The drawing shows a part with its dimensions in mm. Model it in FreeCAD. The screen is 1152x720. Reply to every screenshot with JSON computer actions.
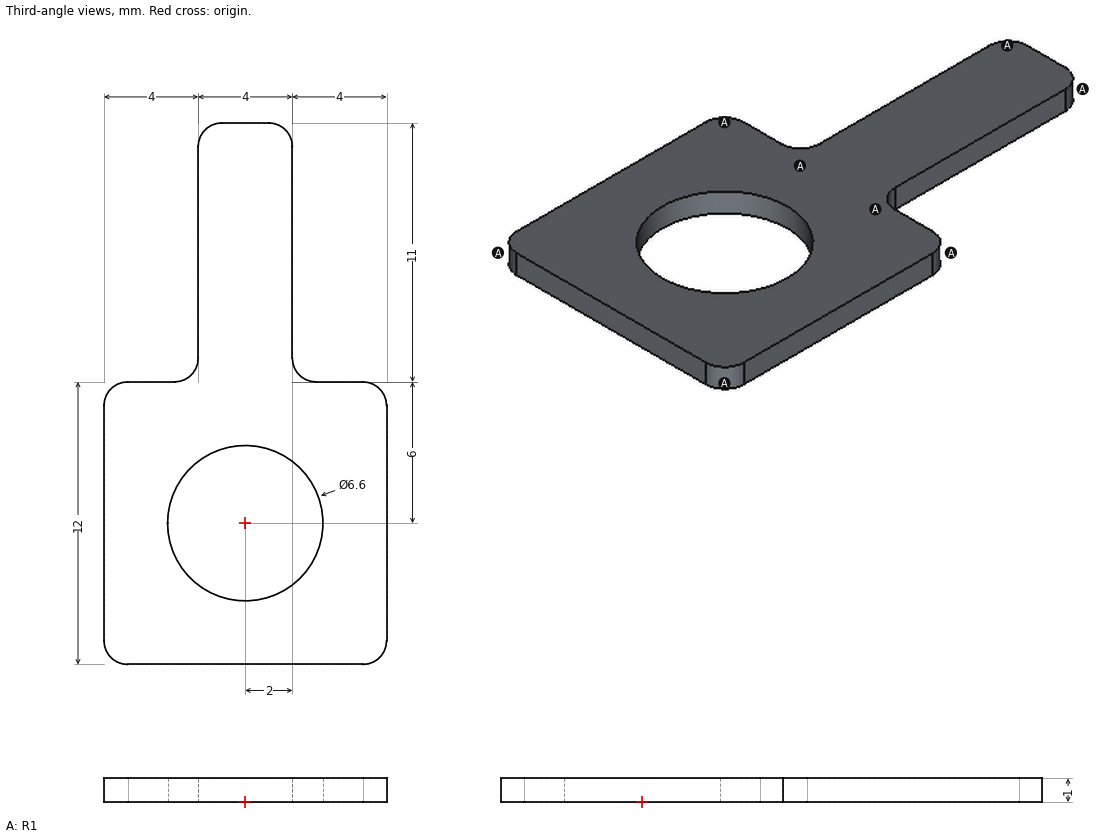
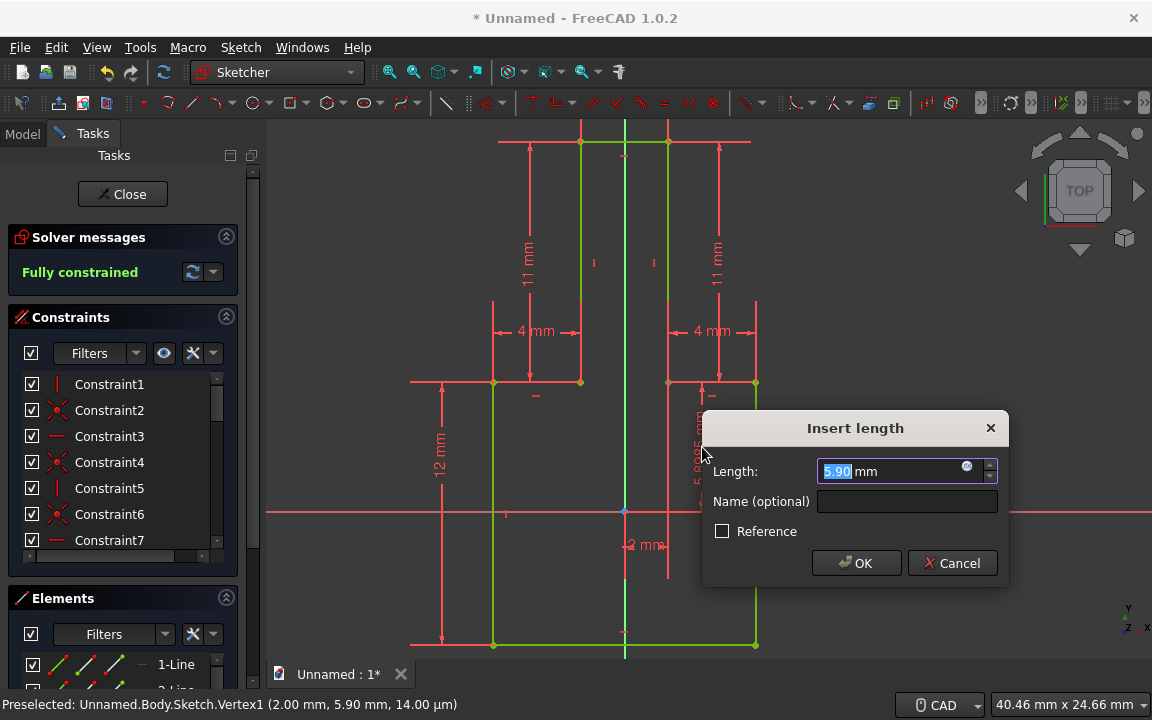
{"action": "type", "text": "6"}
{"action": "key", "text": "Return"}
{"action": "key", "text": "Escape"}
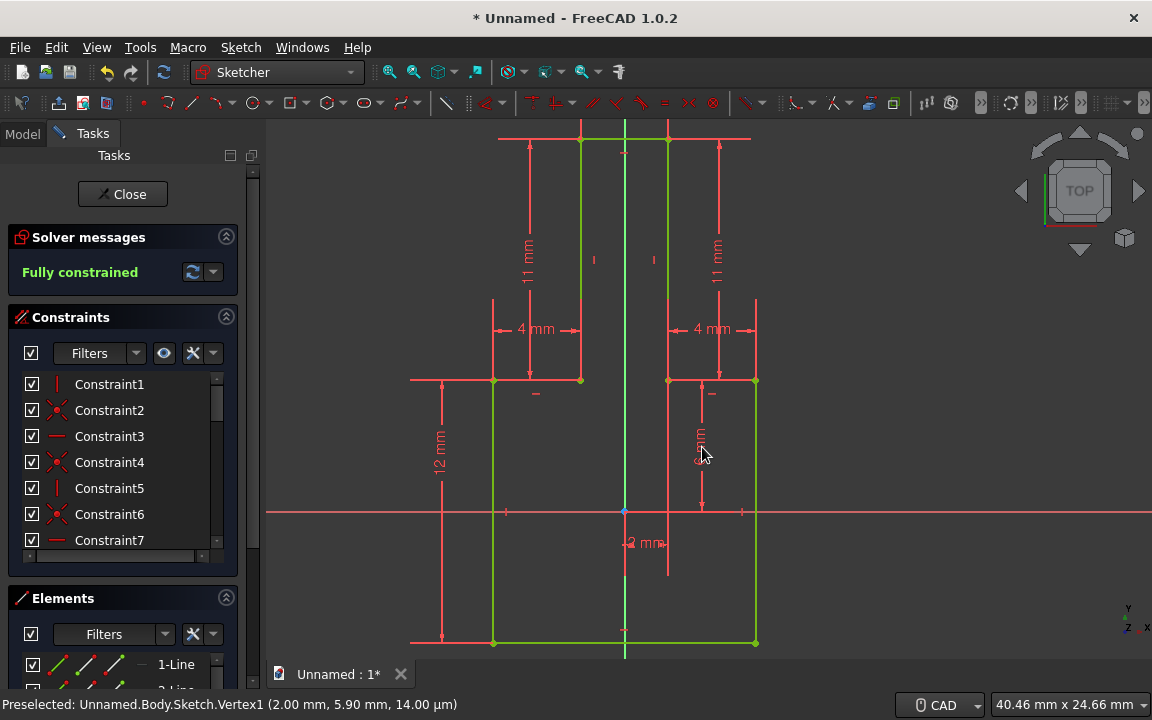
{"action": "left_click", "coordinate": [123, 194]}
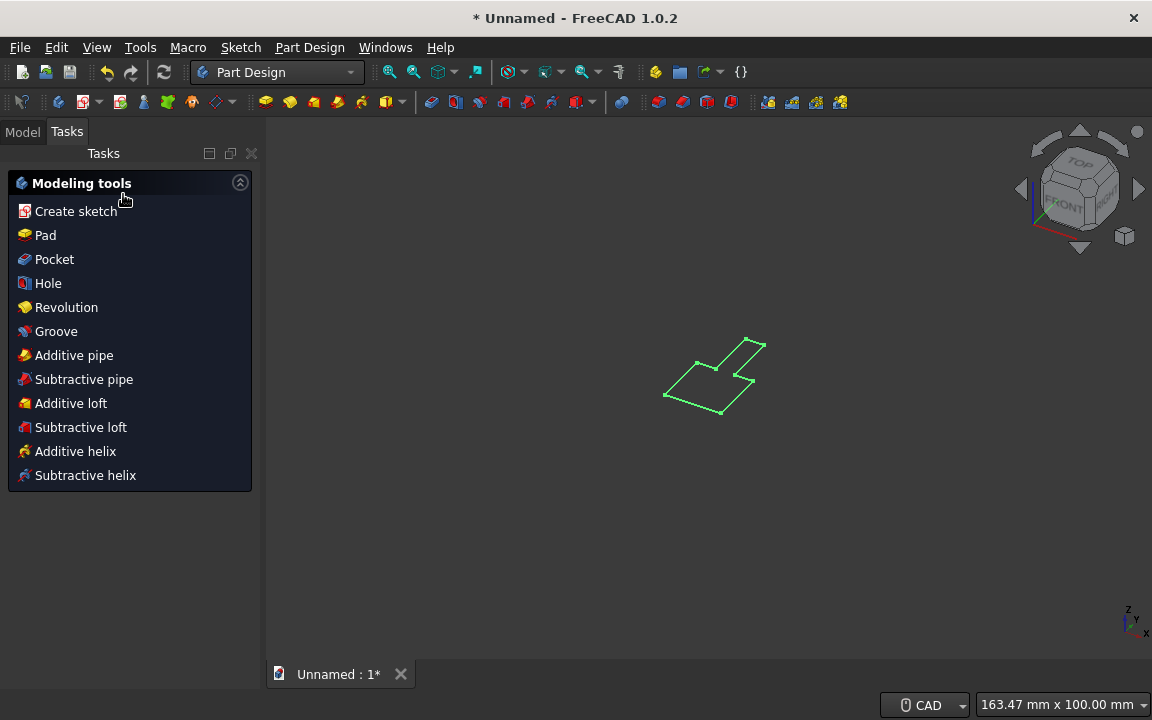
{"action": "left_click", "coordinate": [266, 102]}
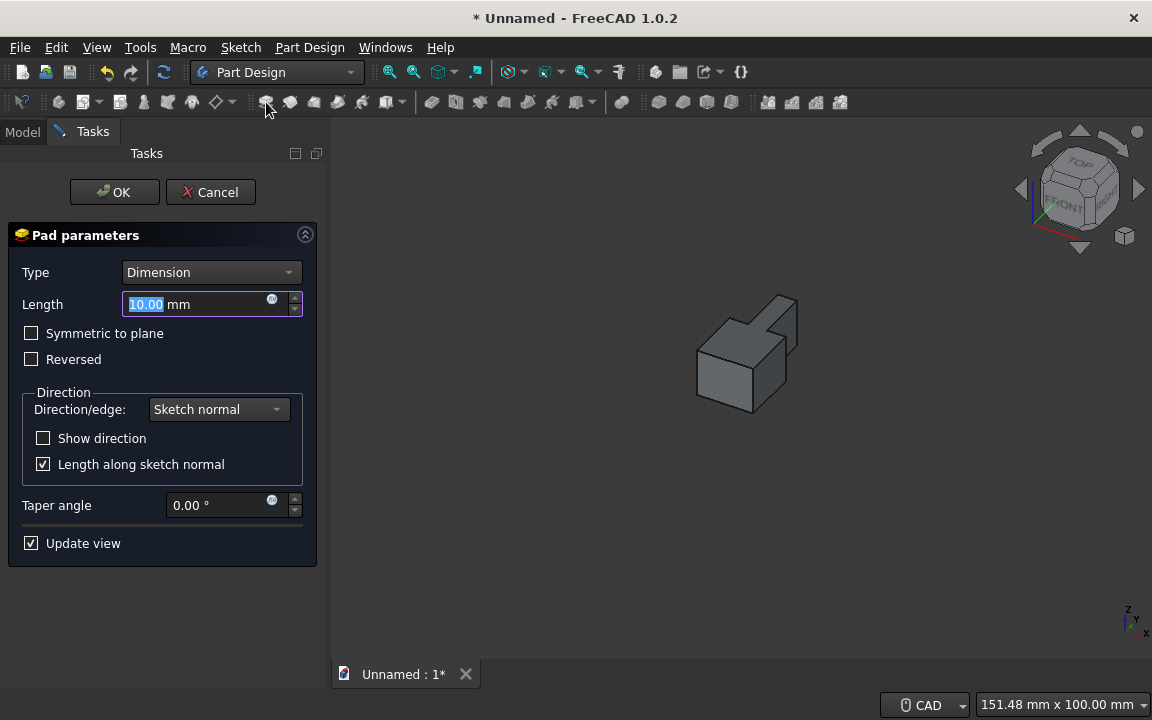
{"action": "type", "text": "1"}
{"action": "key", "text": "Tab"}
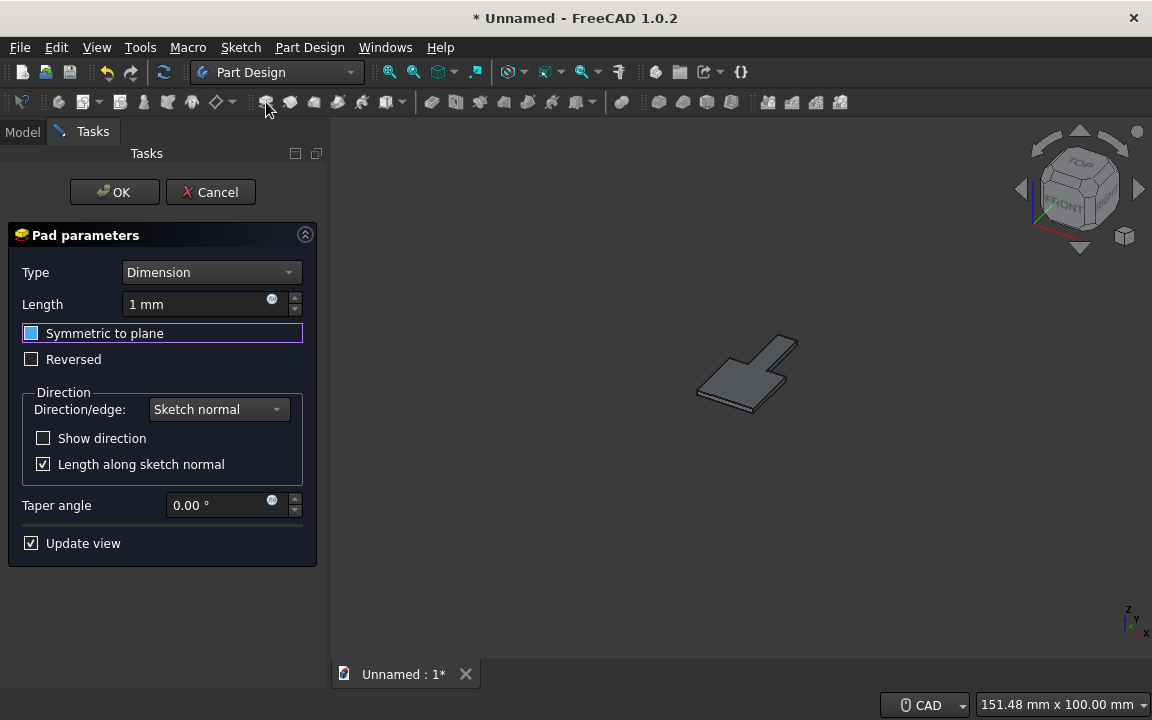
{"action": "left_click", "coordinate": [115, 192]}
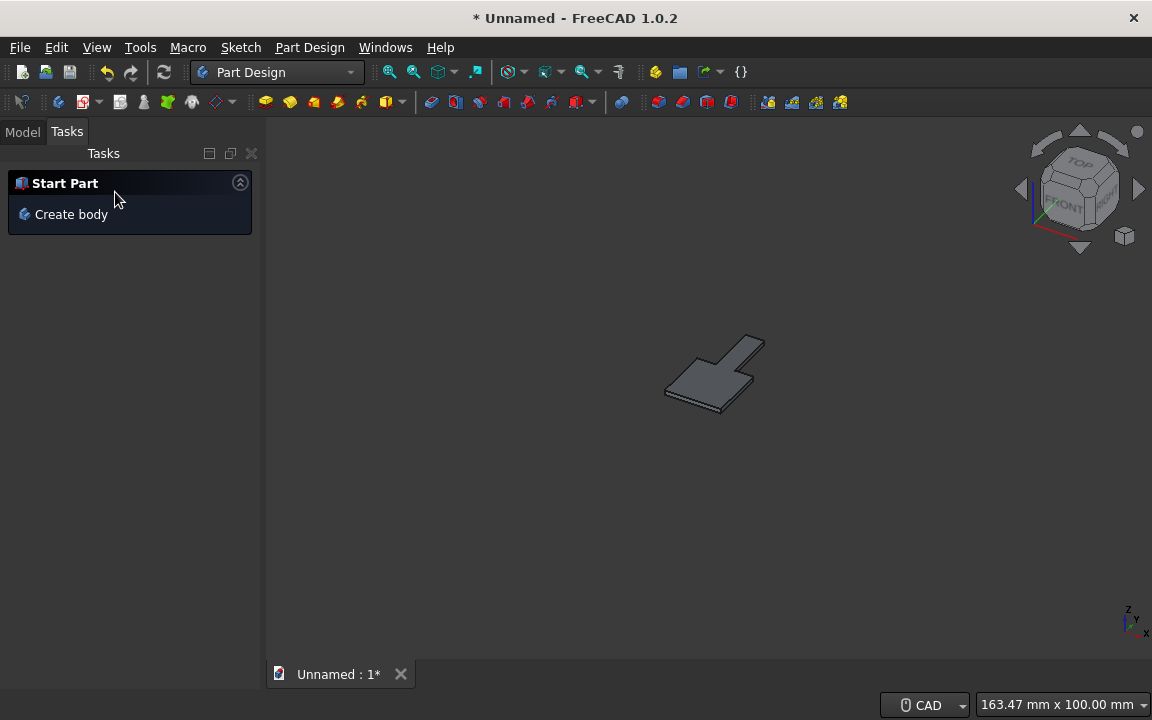
{"action": "key", "text": "v f"}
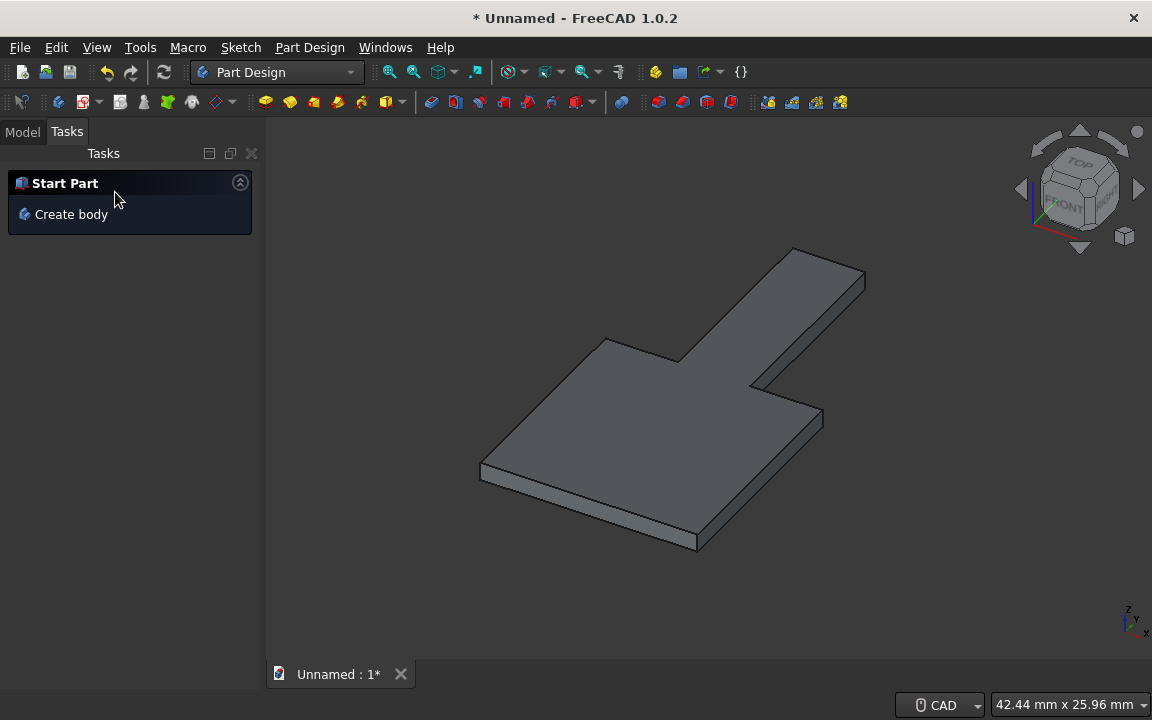
{"action": "left_click", "coordinate": [640, 447]}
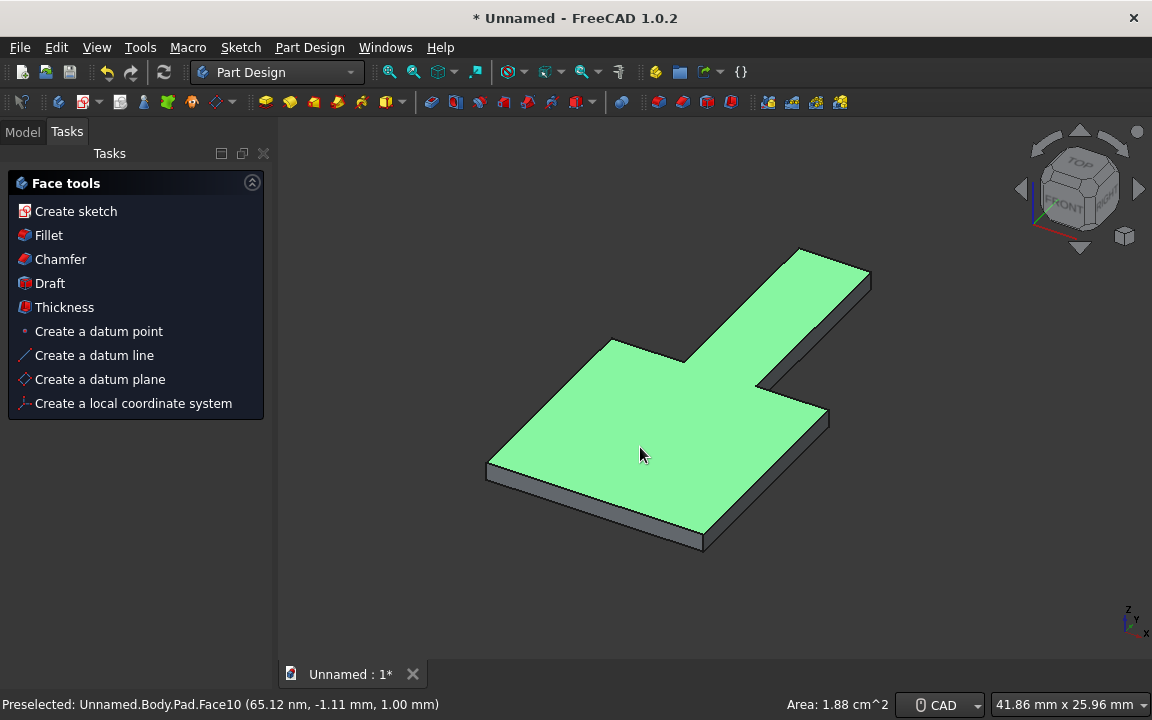
{"action": "left_click", "coordinate": [84, 102]}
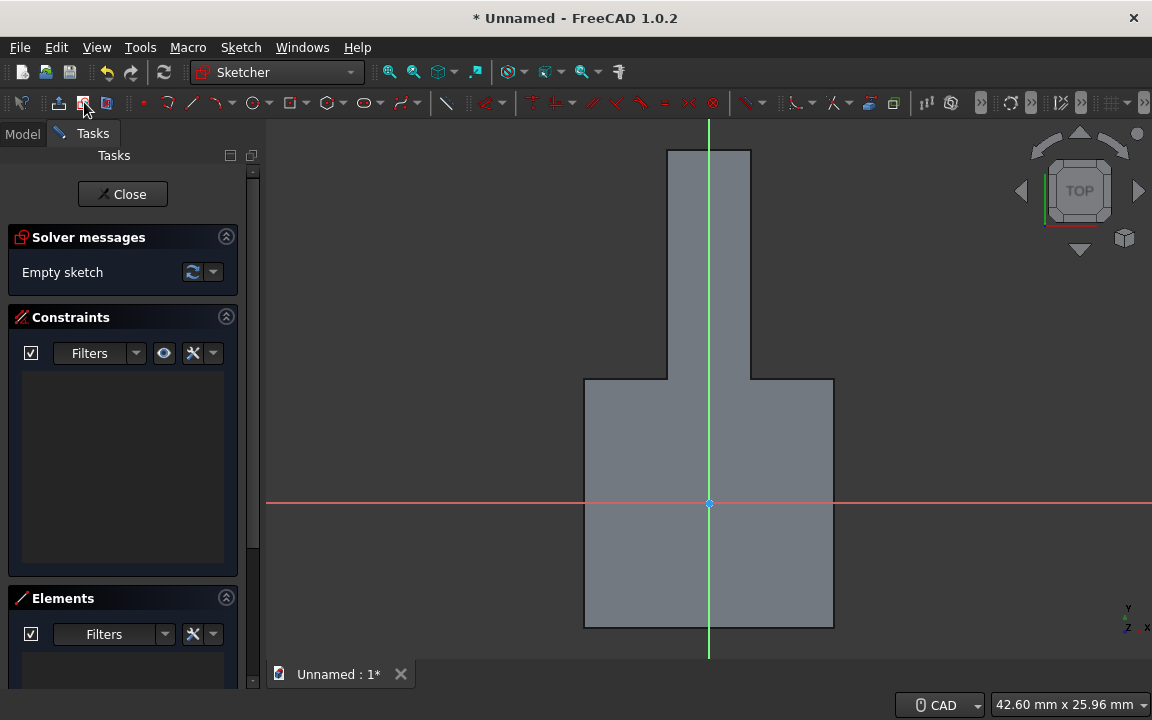
{"action": "scroll", "coordinate": [749, 570], "scroll_direction": "up", "scroll_amount": 5}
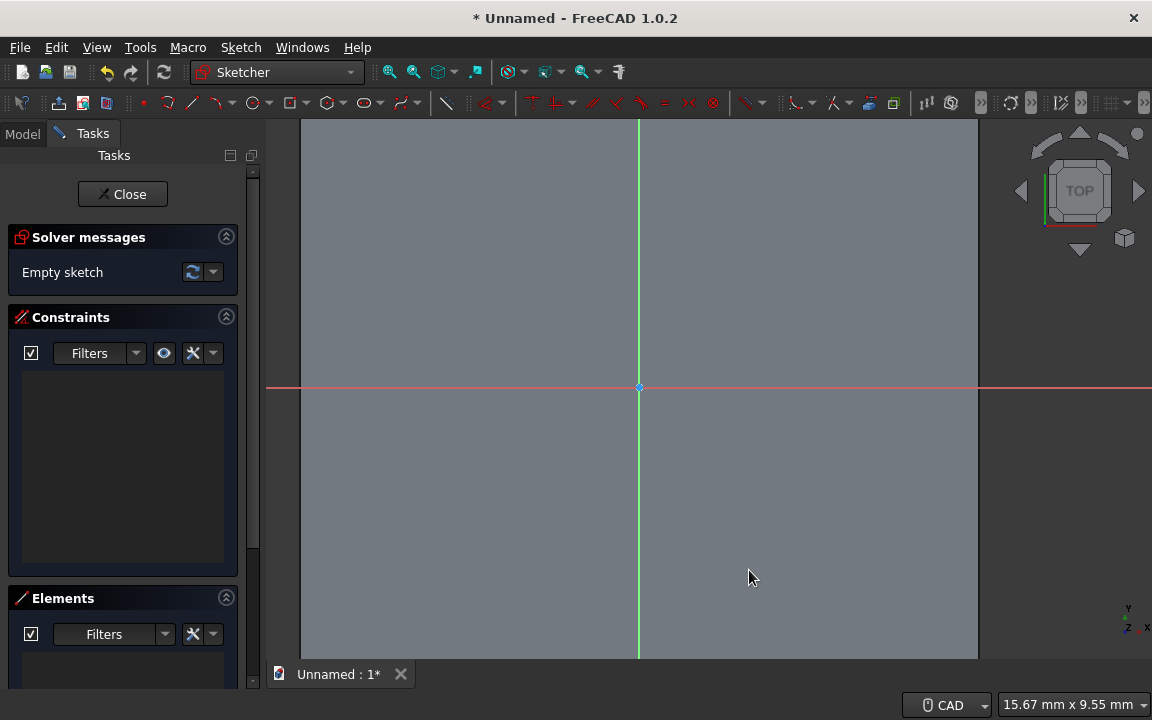
{"action": "key", "text": "g c"}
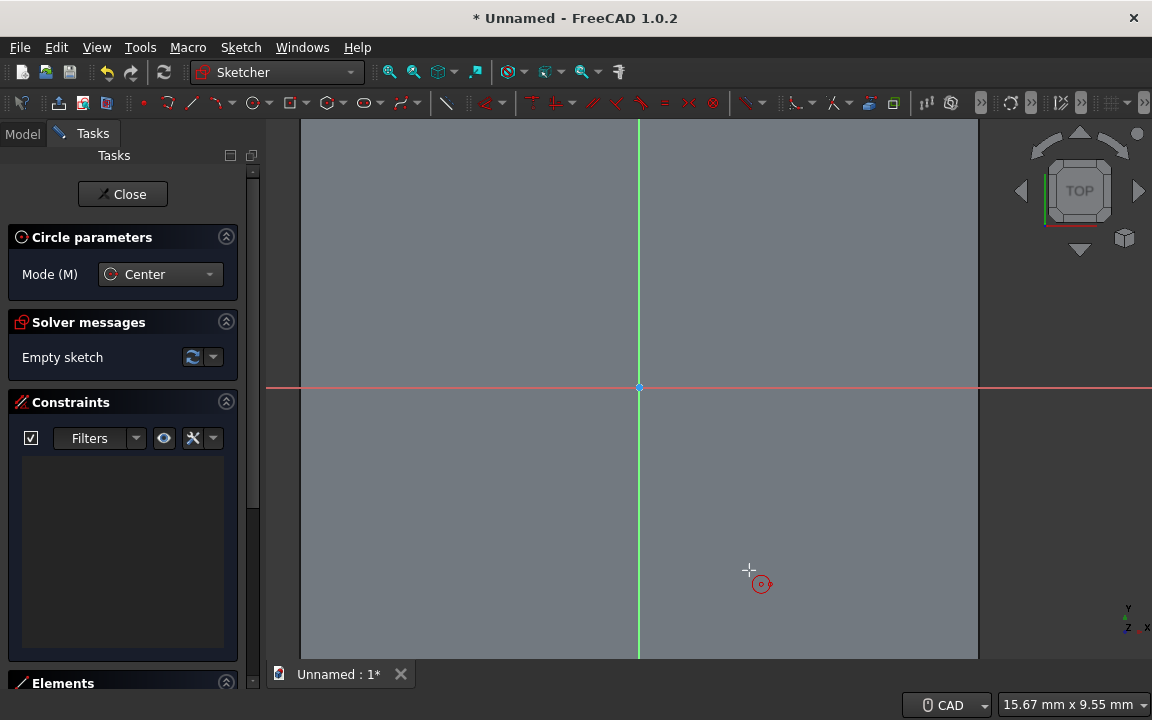
{"action": "left_click", "coordinate": [639, 388]}
{"action": "mouse_move", "coordinate": [771, 256]}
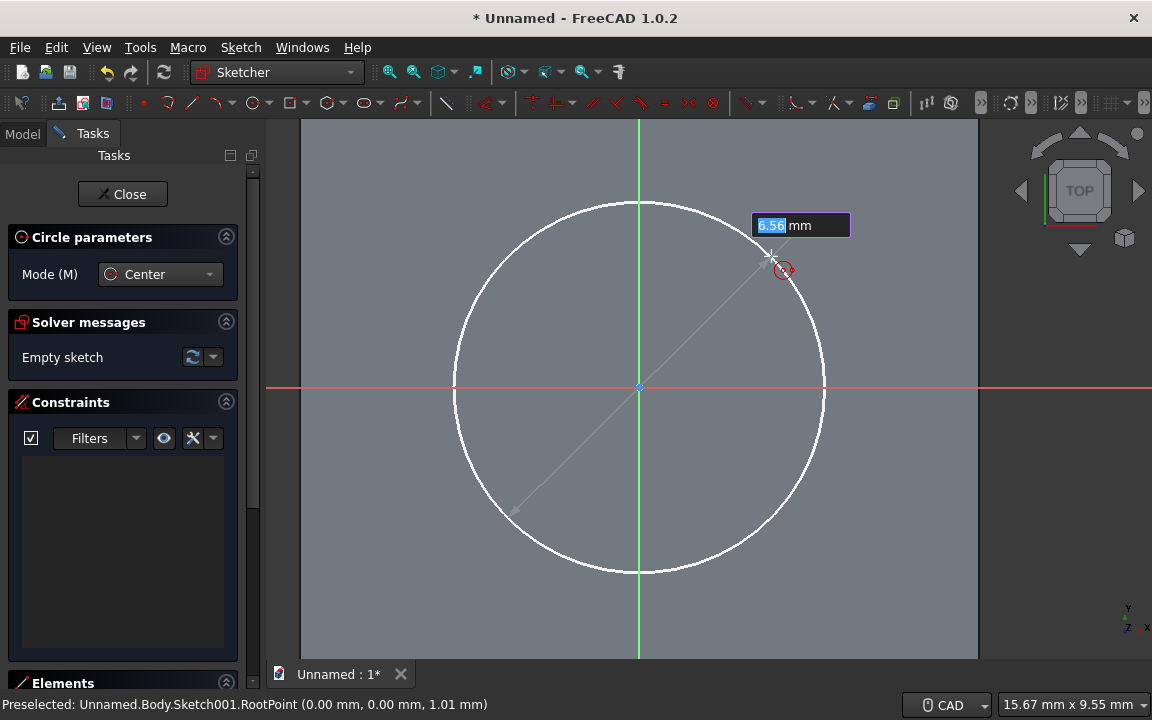
{"action": "type", "text": "6.6"}
{"action": "key", "text": "Return"}
{"action": "key", "text": "Escape"}